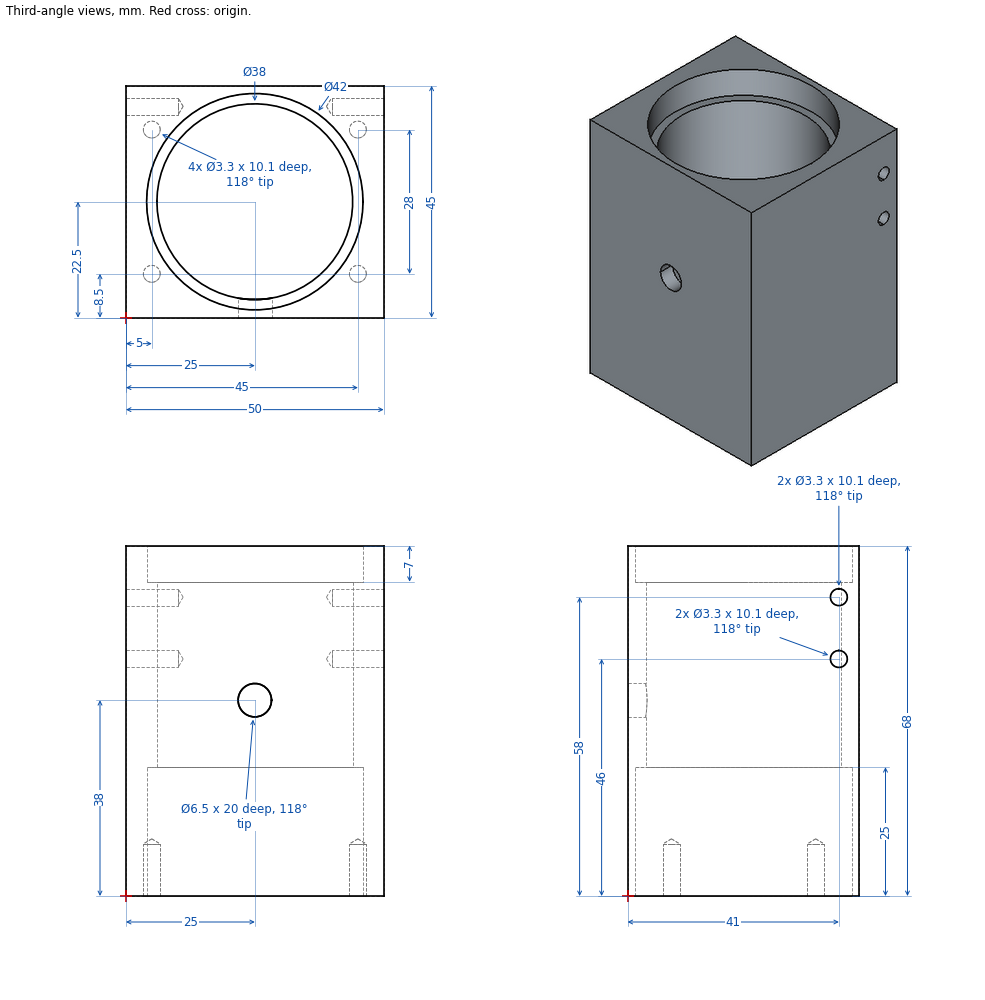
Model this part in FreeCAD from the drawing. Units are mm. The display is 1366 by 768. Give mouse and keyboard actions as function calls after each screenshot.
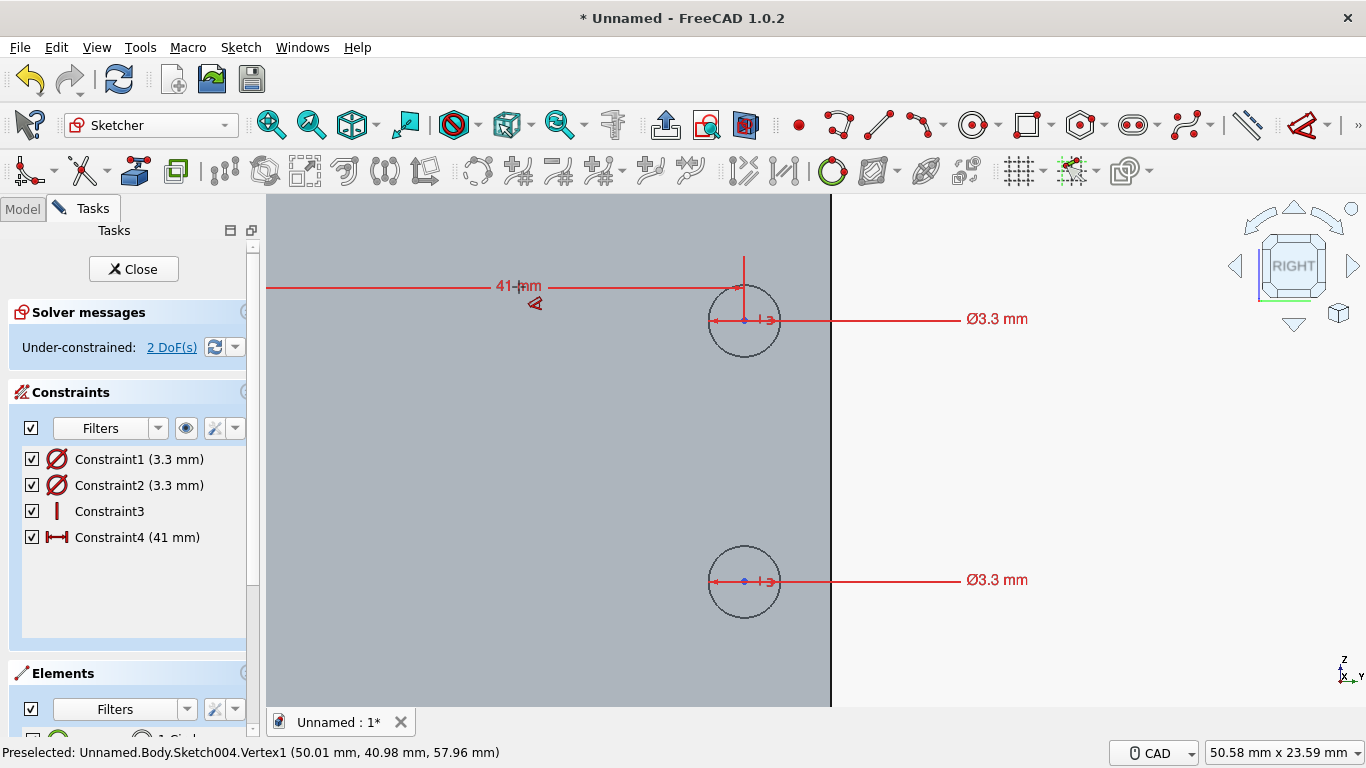
click(744, 321)
click(778, 500)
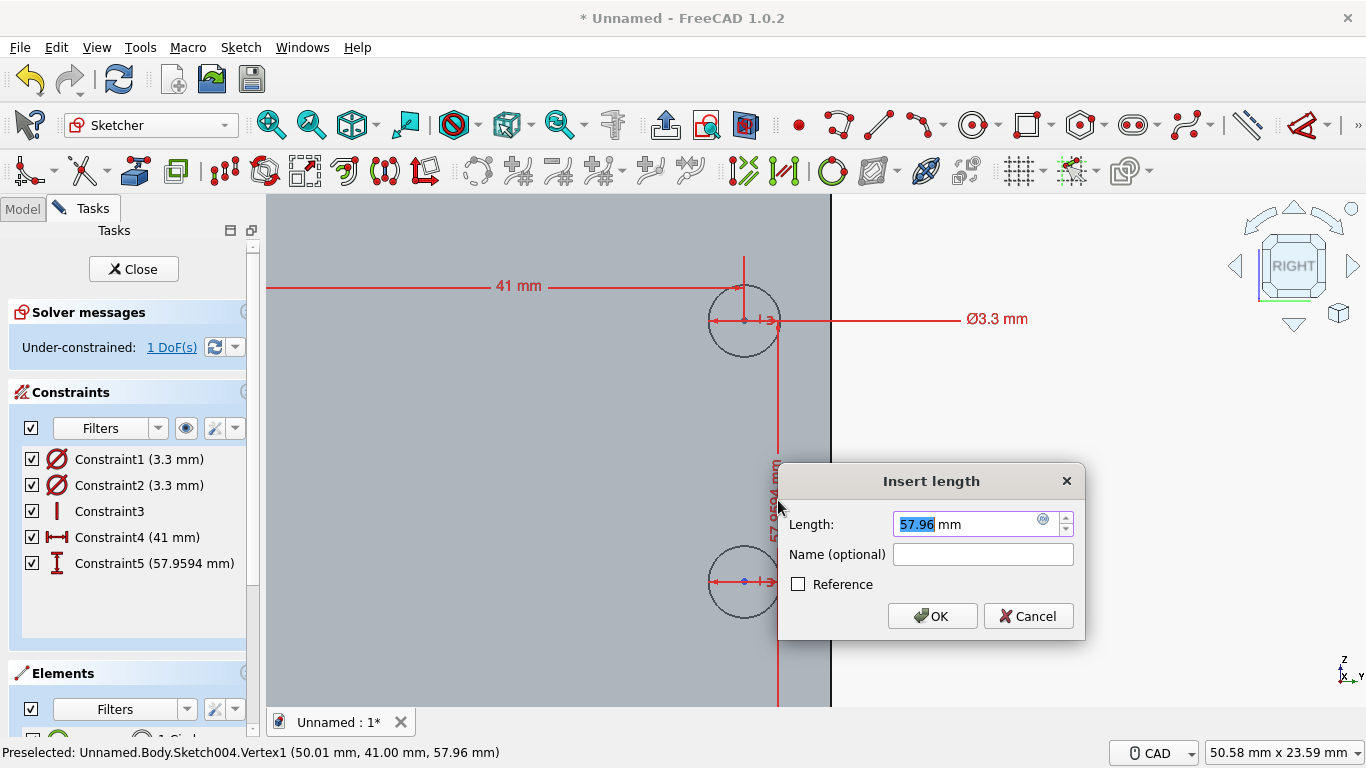
text(58)
key(Return)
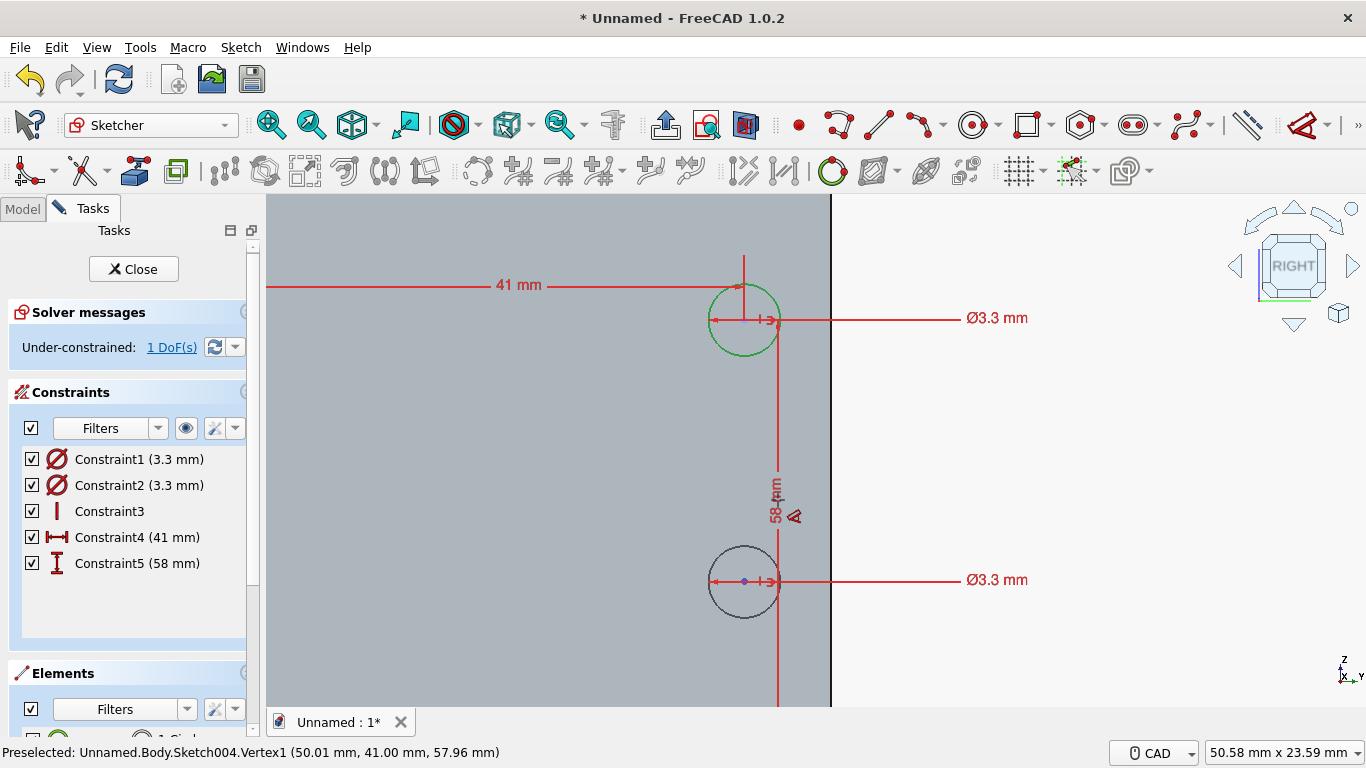
click(744, 582)
click(778, 631)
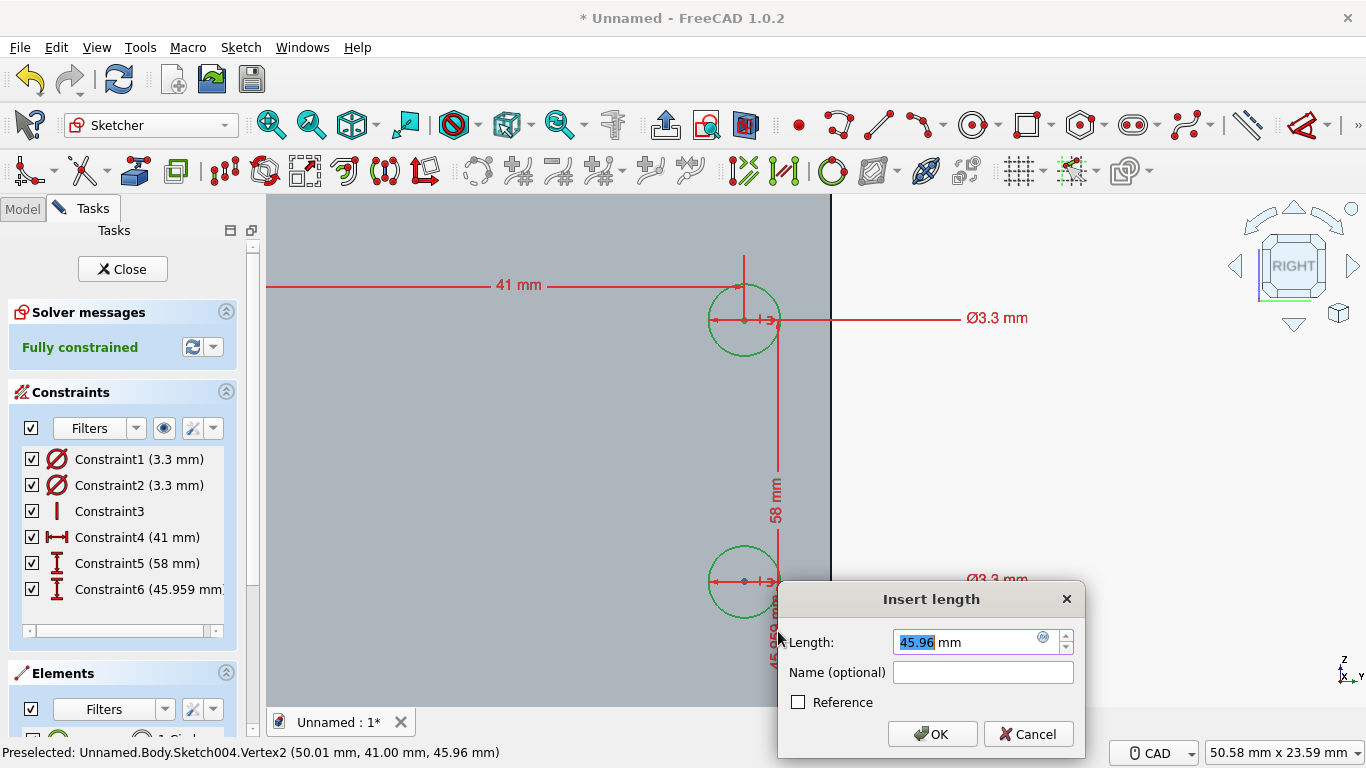
text(46)
key(Return)
key(Escape)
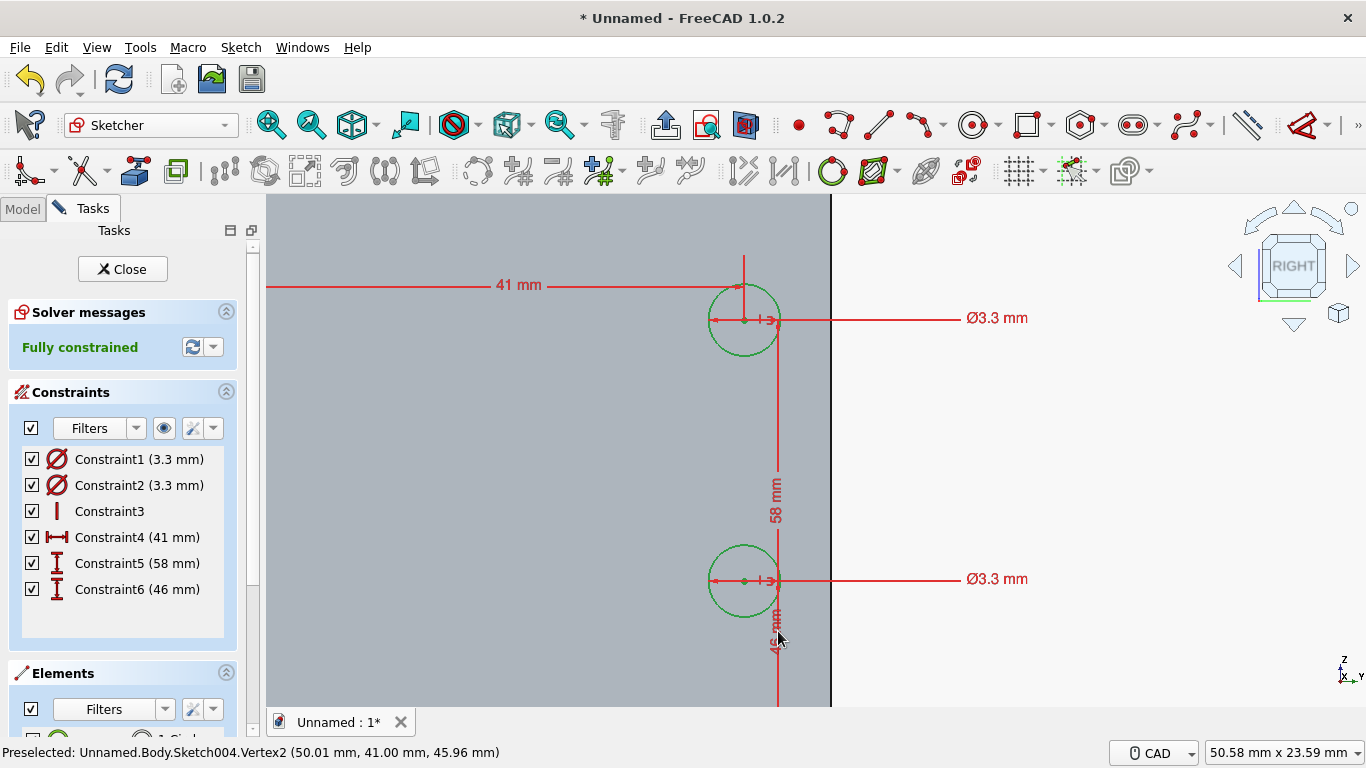
click(123, 269)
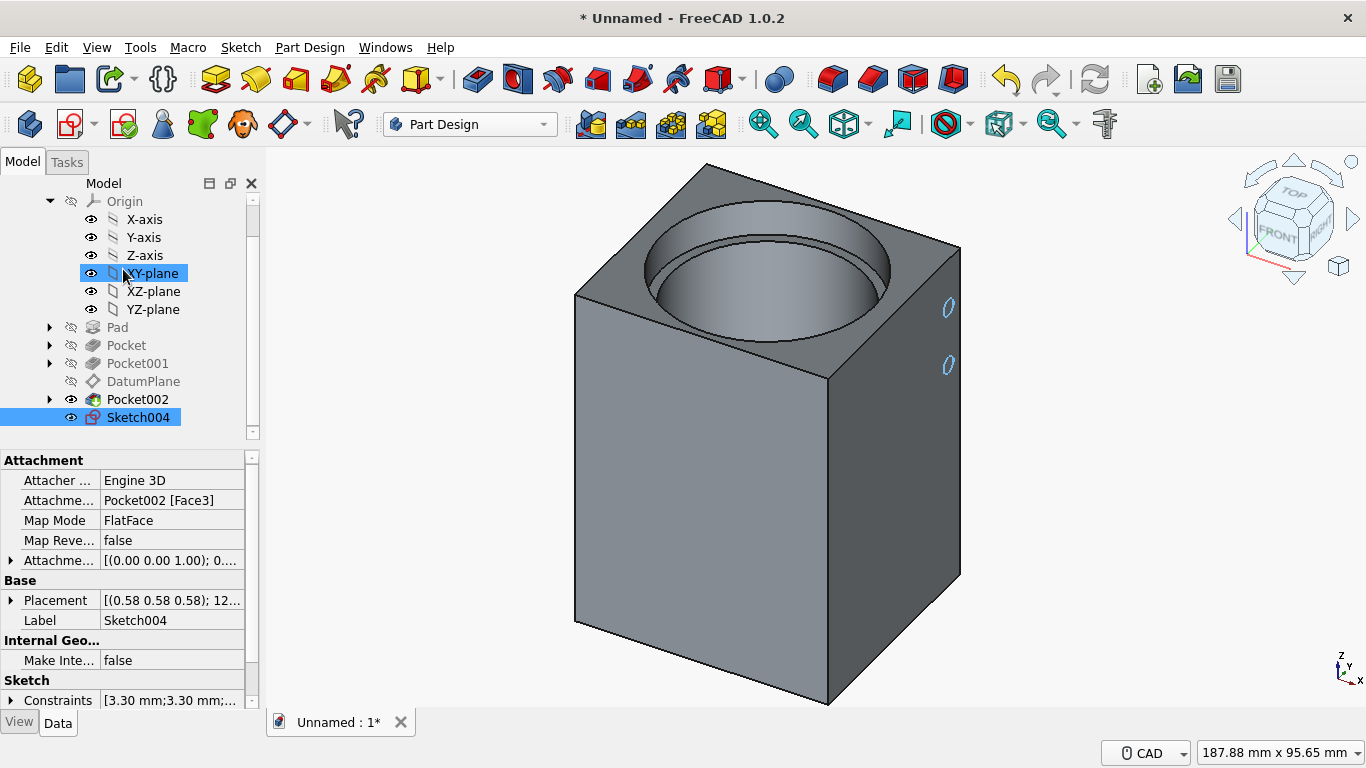
click(518, 80)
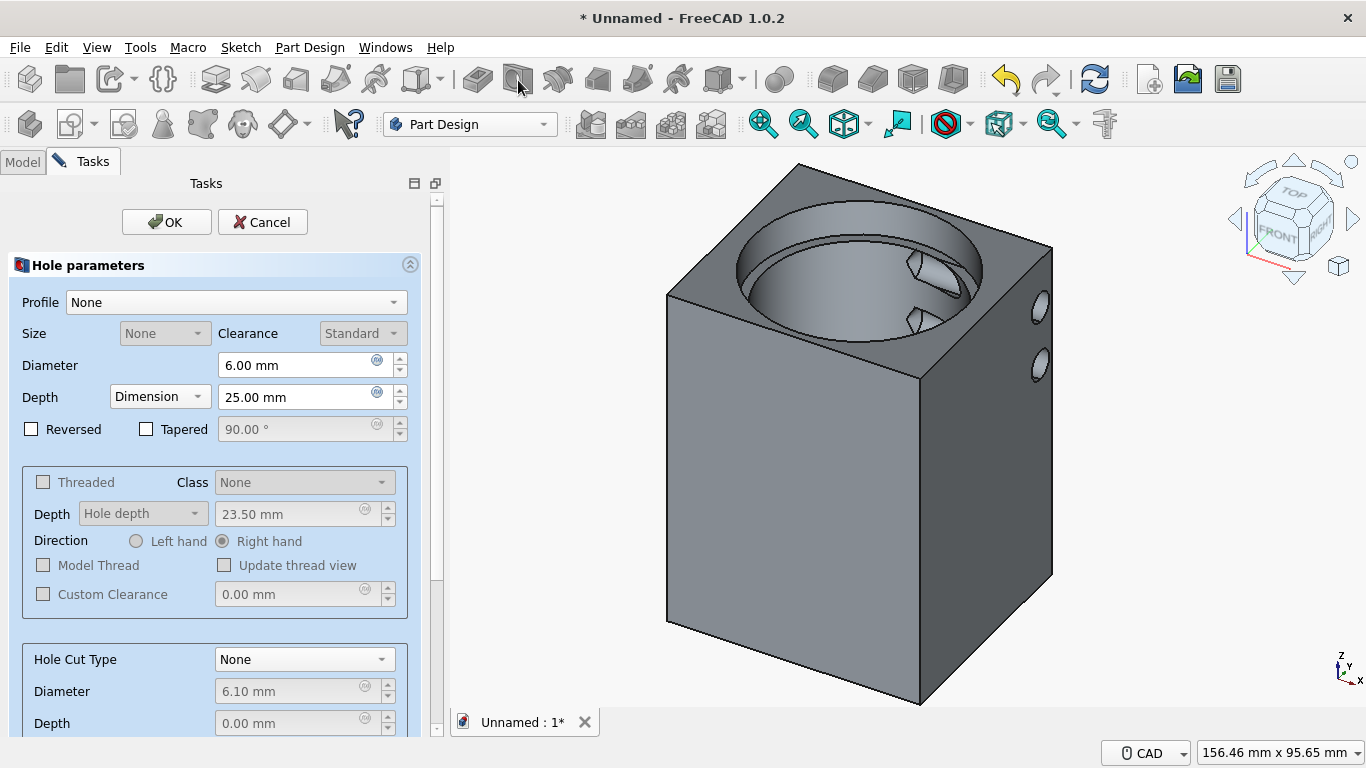
triple_click(305, 365)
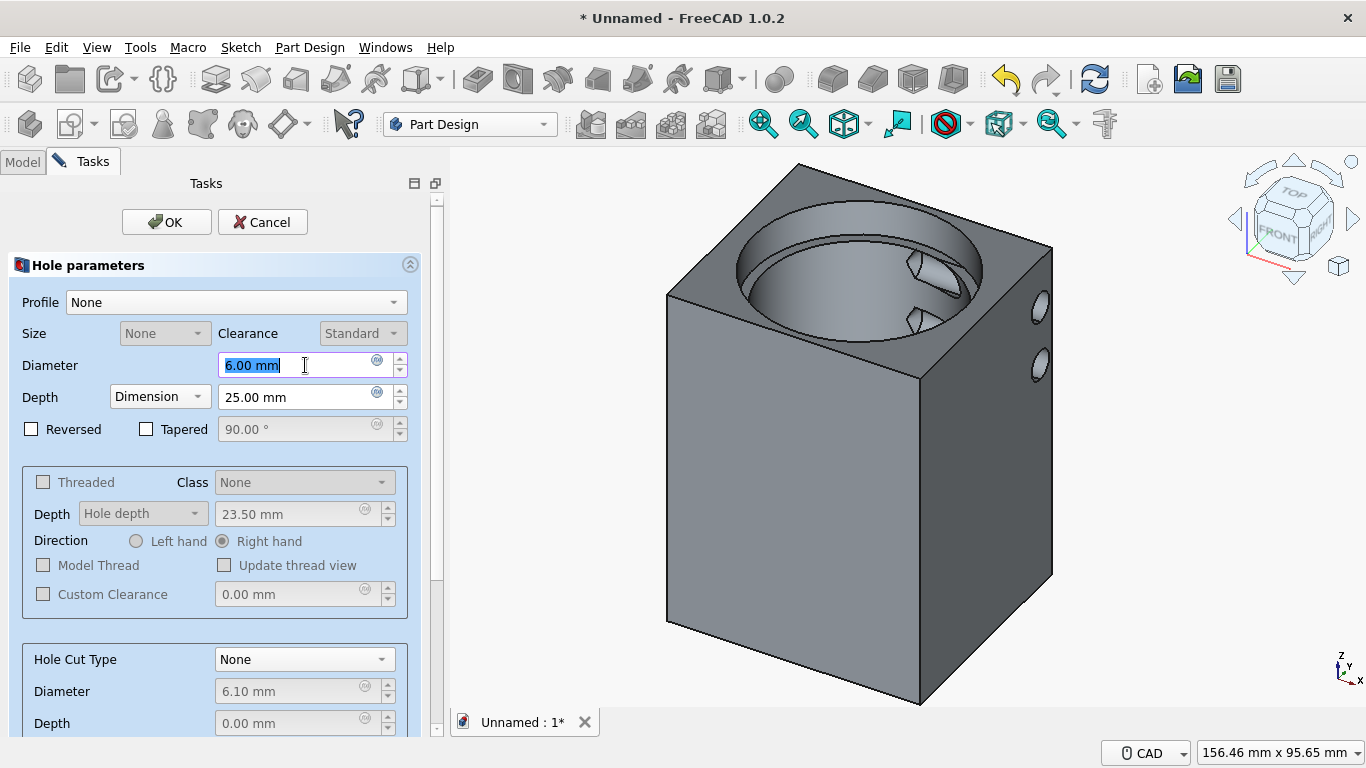
text(3.3)
key(Tab)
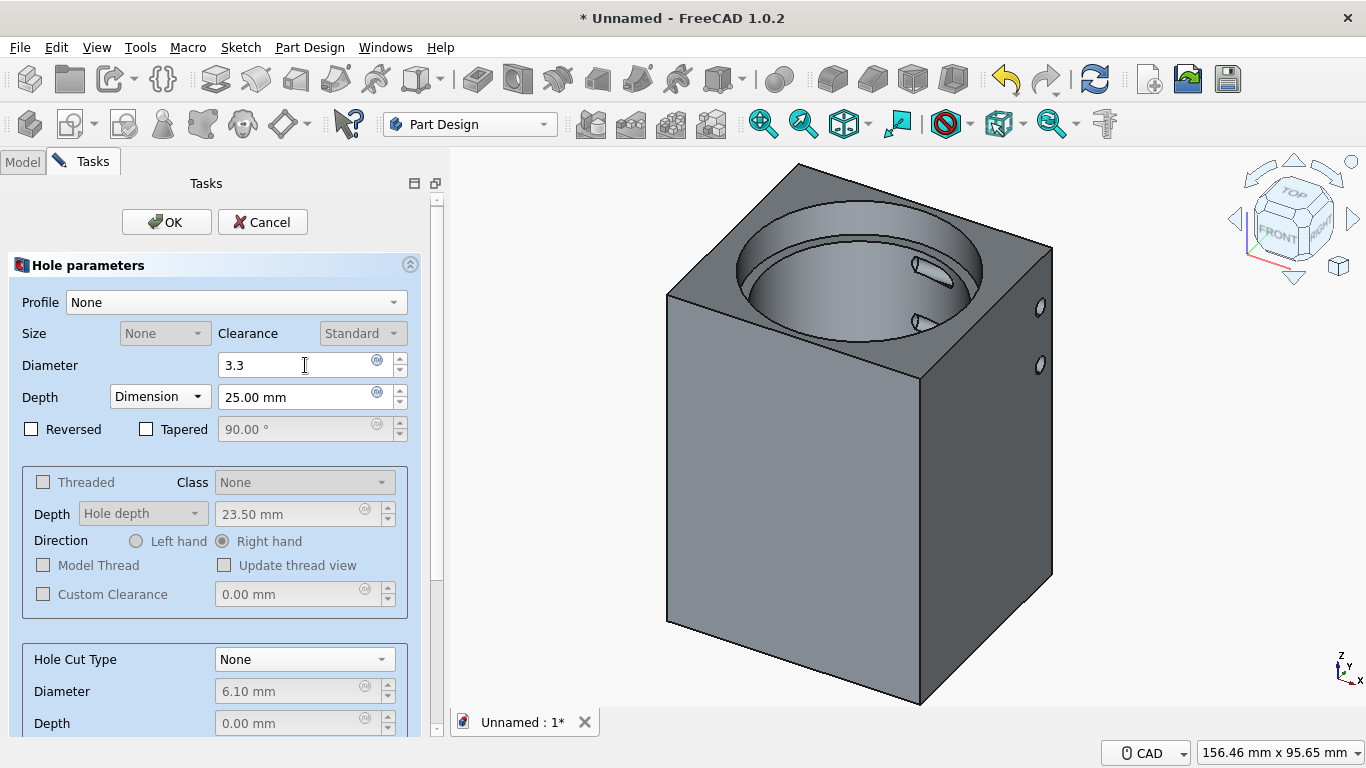
triple_click(305, 397)